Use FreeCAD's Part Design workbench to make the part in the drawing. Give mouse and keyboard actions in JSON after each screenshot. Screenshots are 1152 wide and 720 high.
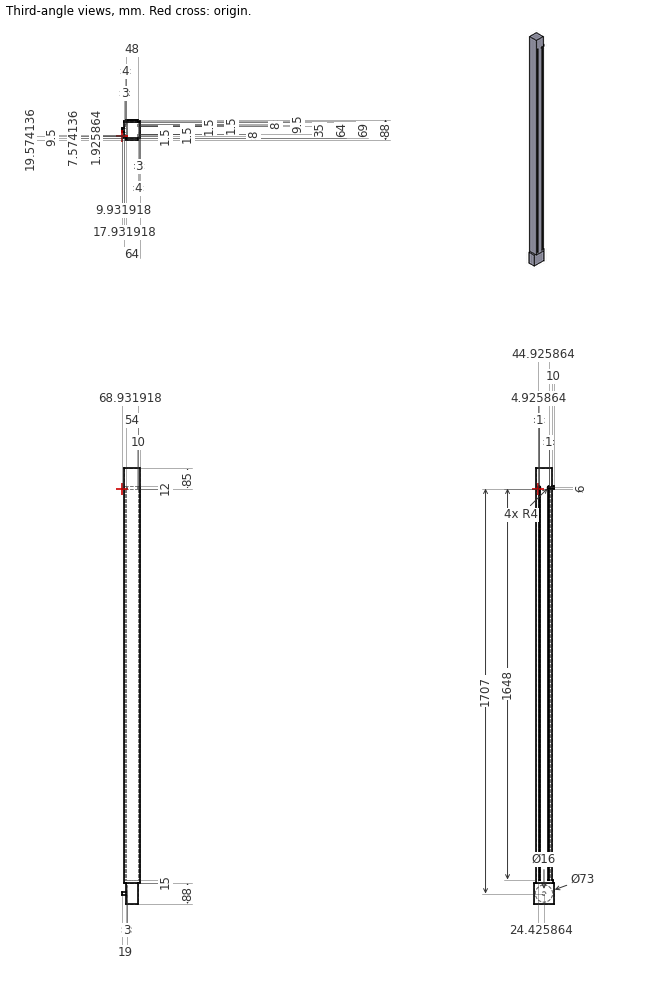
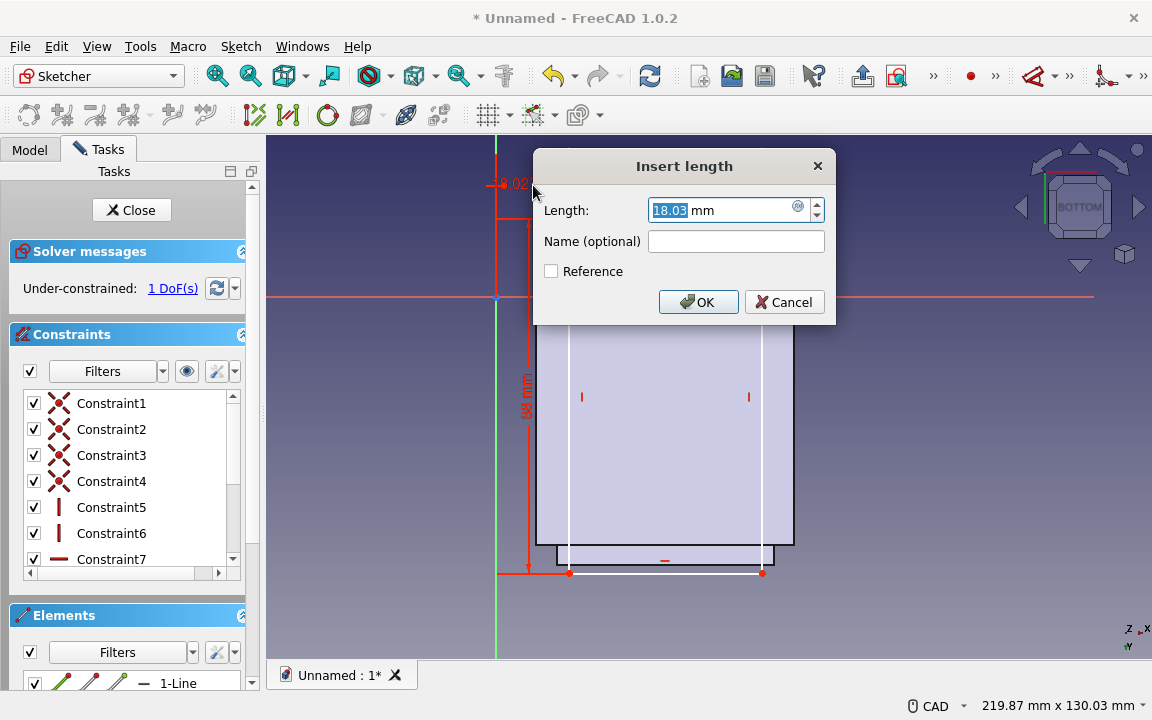
{"action": "type", "text": "17.931918"}
{"action": "key", "text": "Return"}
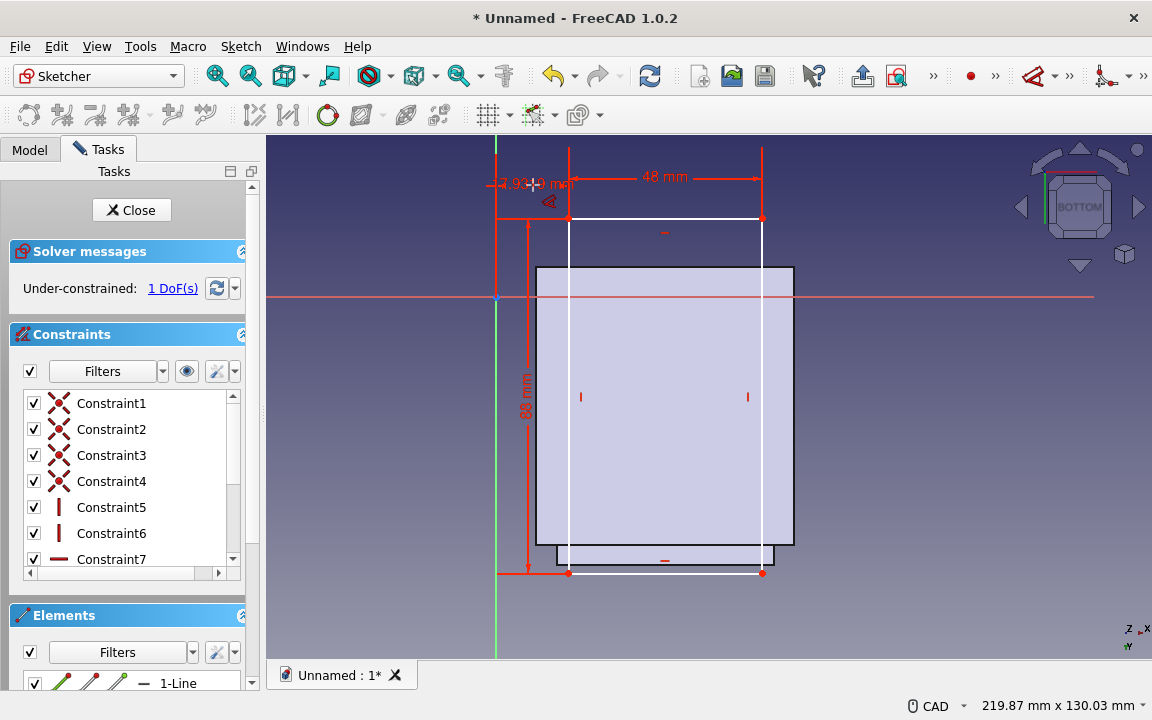
{"action": "left_click", "coordinate": [569, 219]}
{"action": "left_click", "coordinate": [462, 258]}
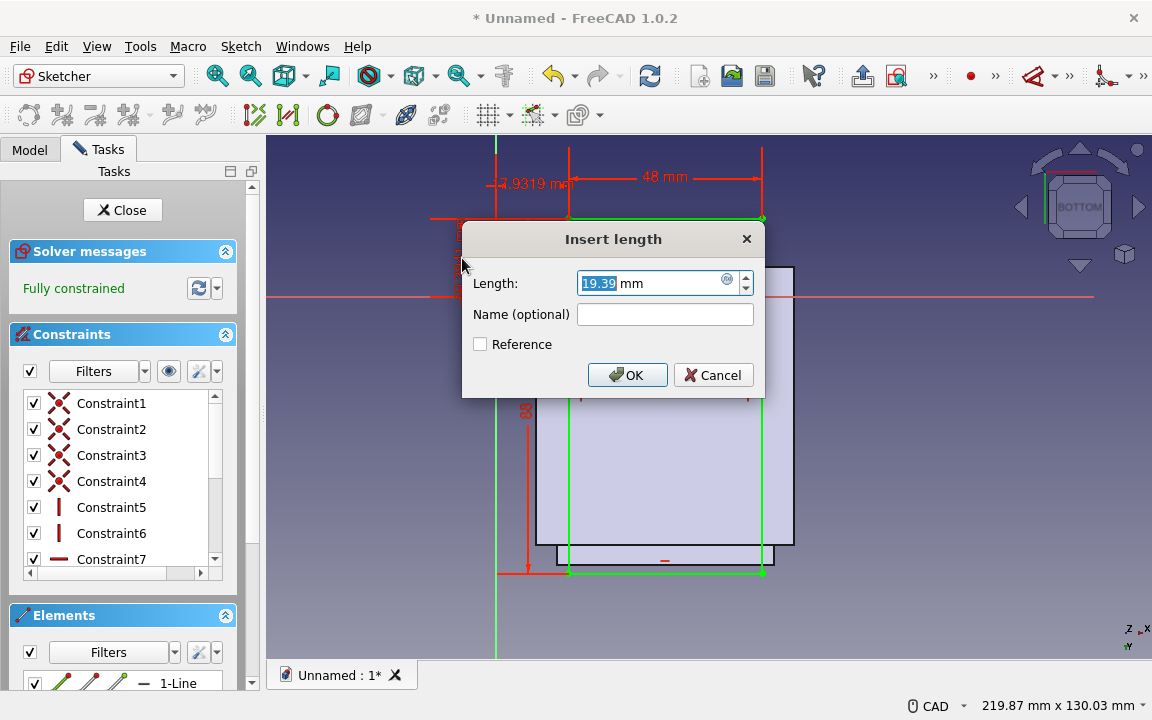
{"action": "type", "text": "19.574136"}
{"action": "key", "text": "Return"}
{"action": "key", "text": "Escape"}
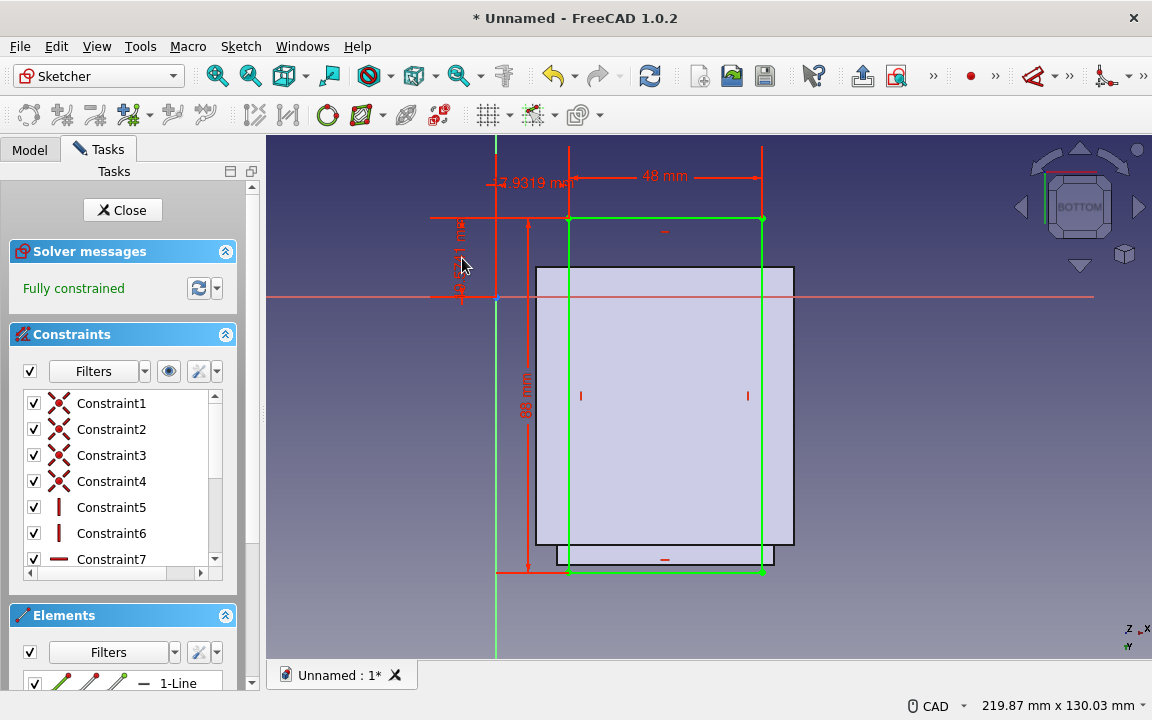
{"action": "left_click", "coordinate": [123, 210]}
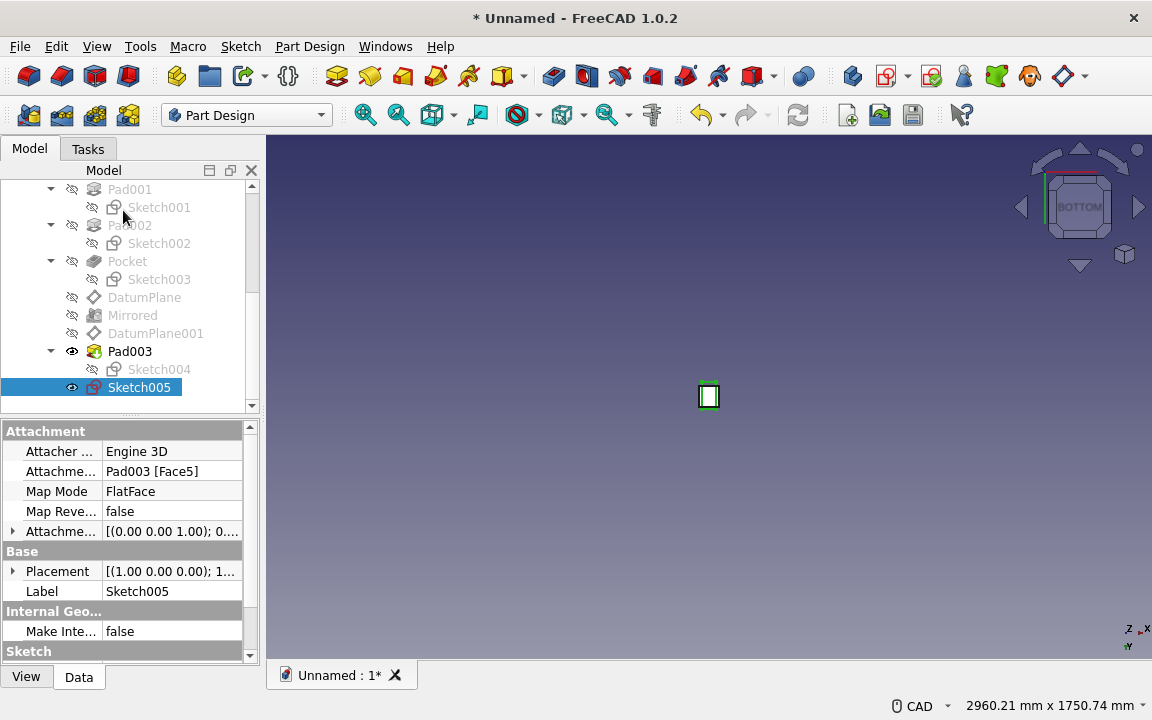
{"action": "left_click", "coordinate": [337, 76]}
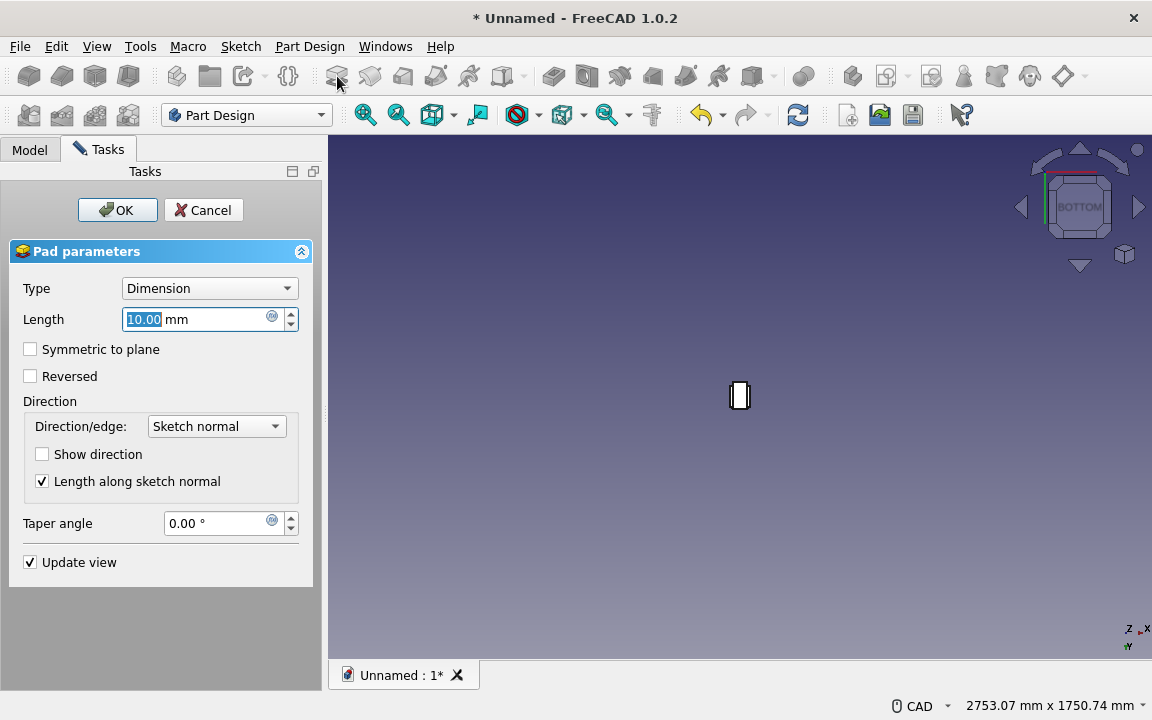
{"action": "type", "text": "88"}
{"action": "key", "text": "Tab"}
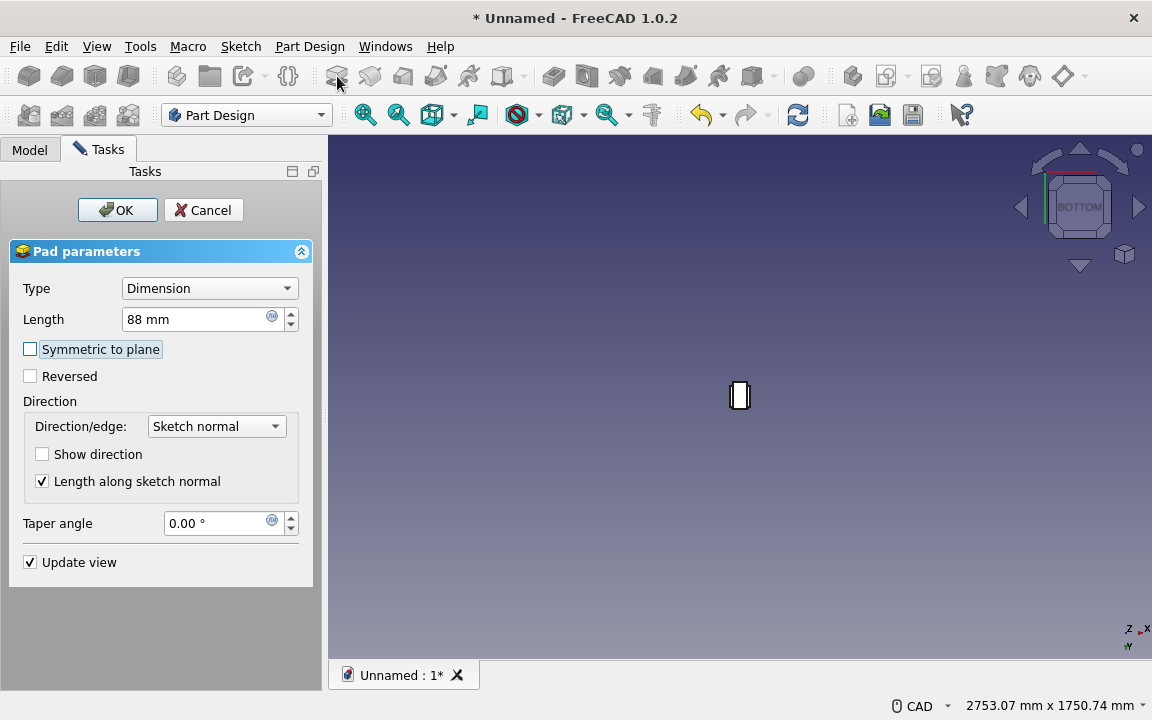
{"action": "left_click", "coordinate": [118, 210]}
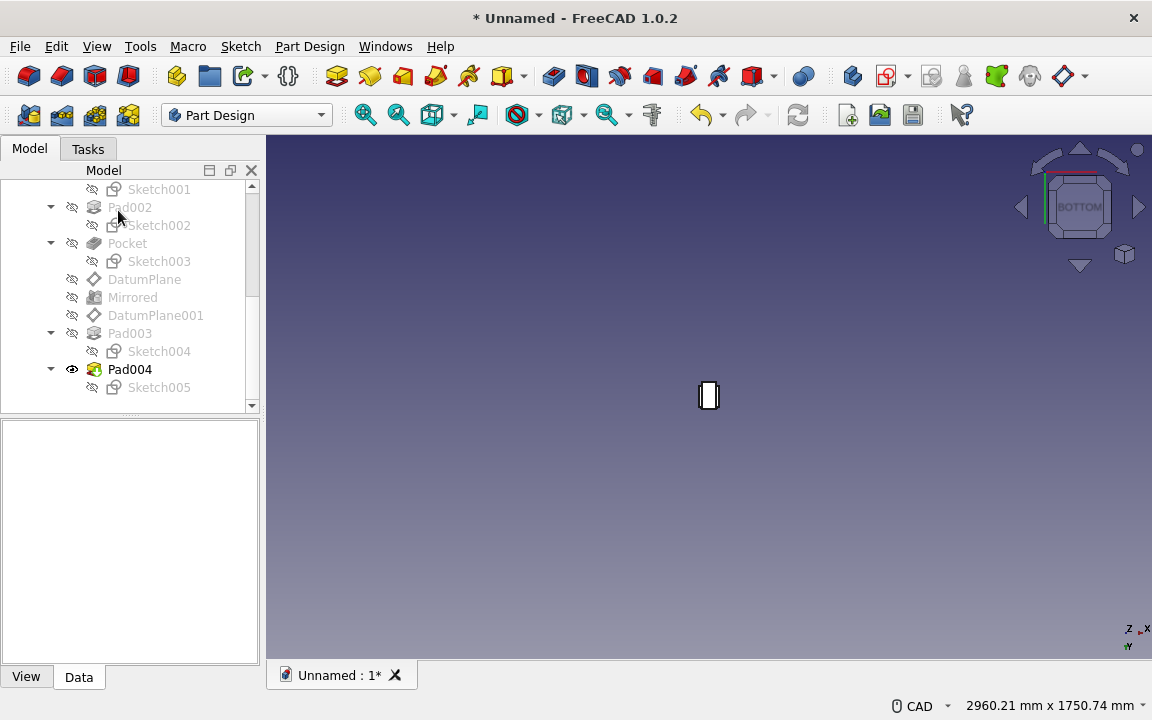
{"action": "left_click", "coordinate": [366, 116]}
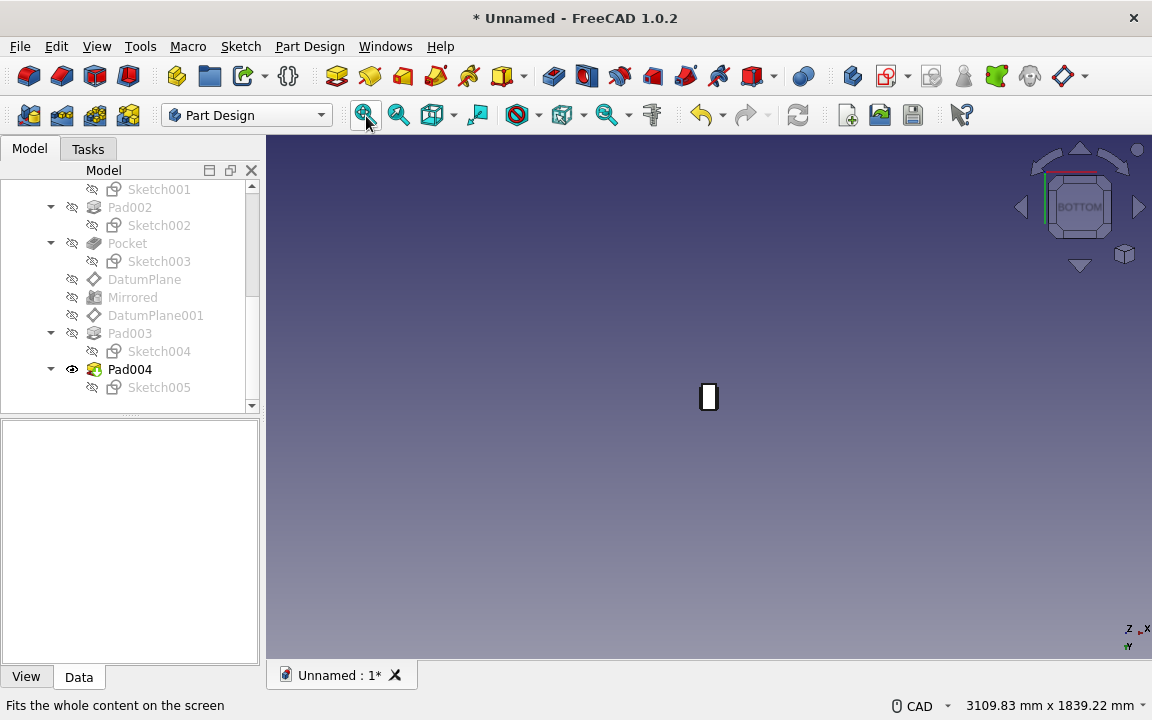
{"action": "key", "text": "6"}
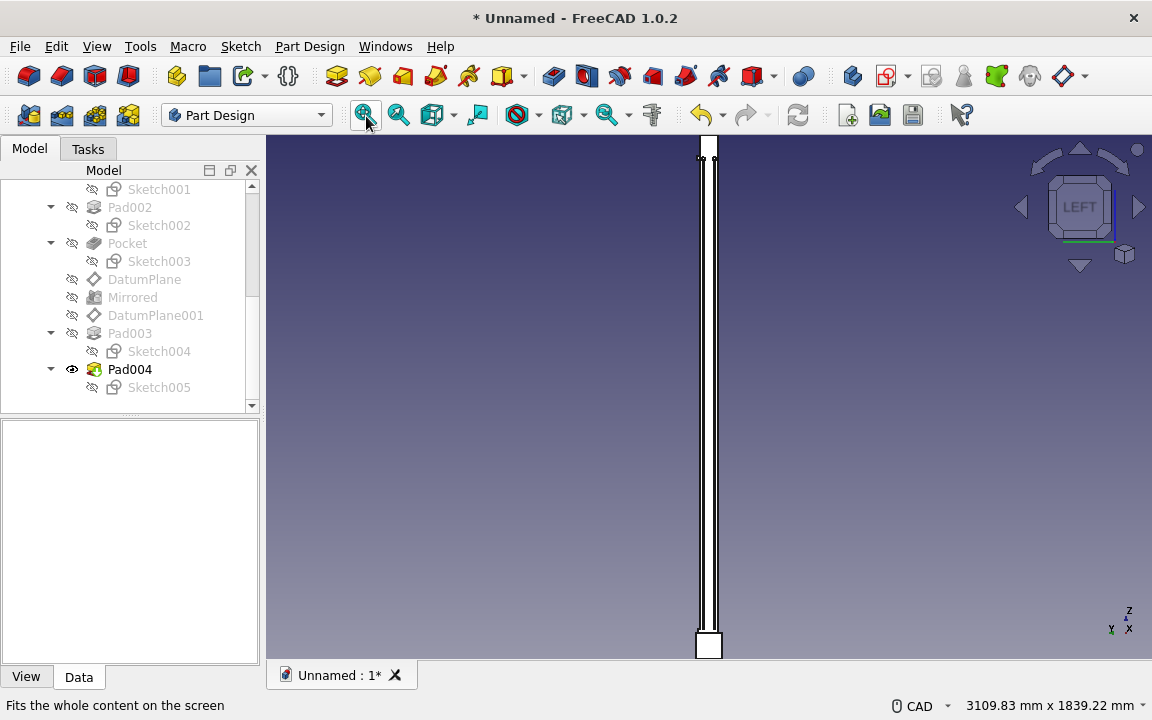
{"action": "left_click", "coordinate": [366, 116]}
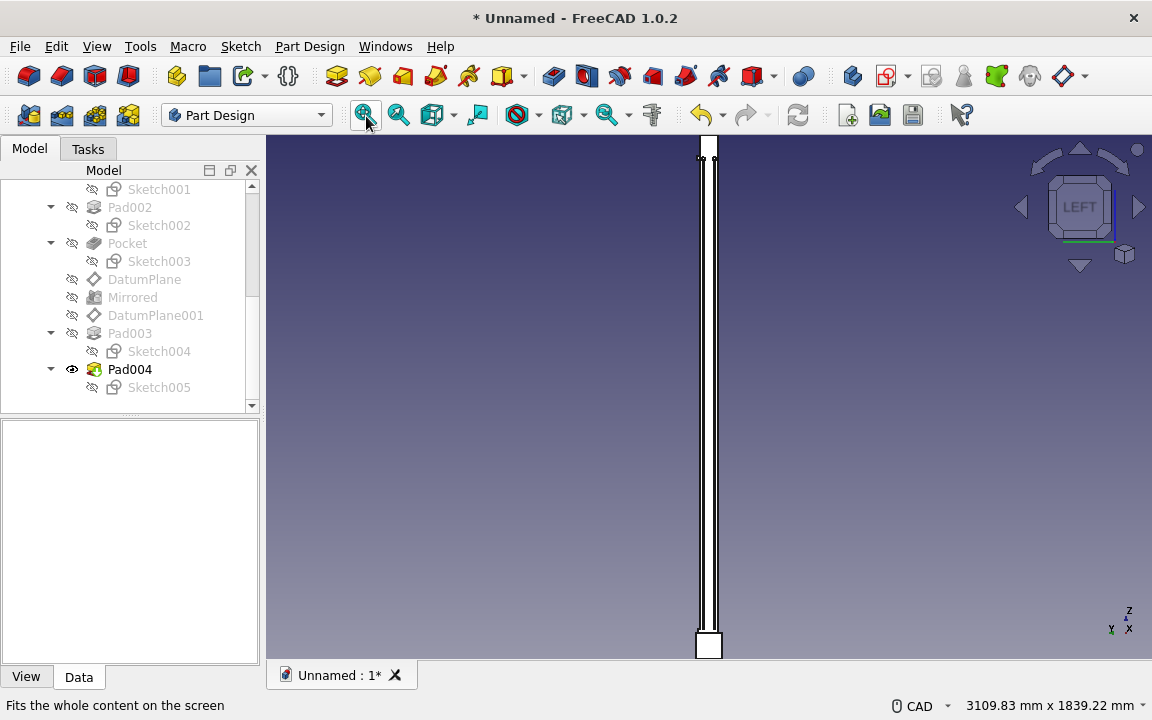
{"action": "key", "text": "2"}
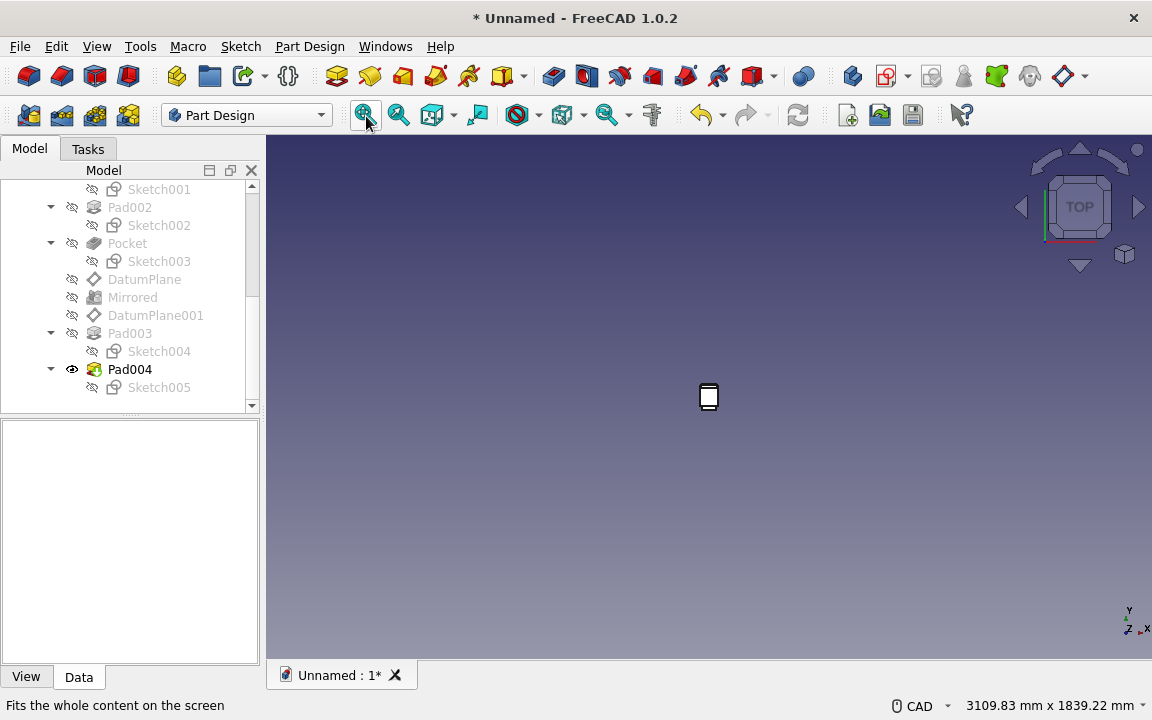
{"action": "left_click", "coordinate": [366, 116]}